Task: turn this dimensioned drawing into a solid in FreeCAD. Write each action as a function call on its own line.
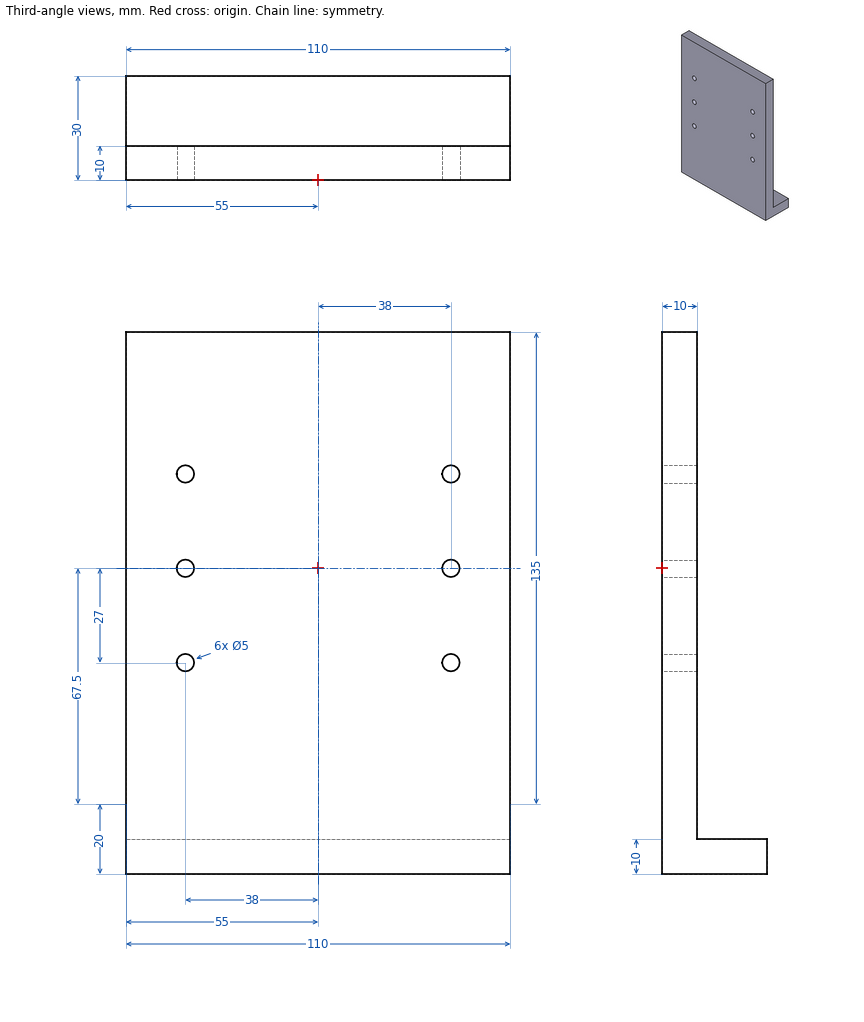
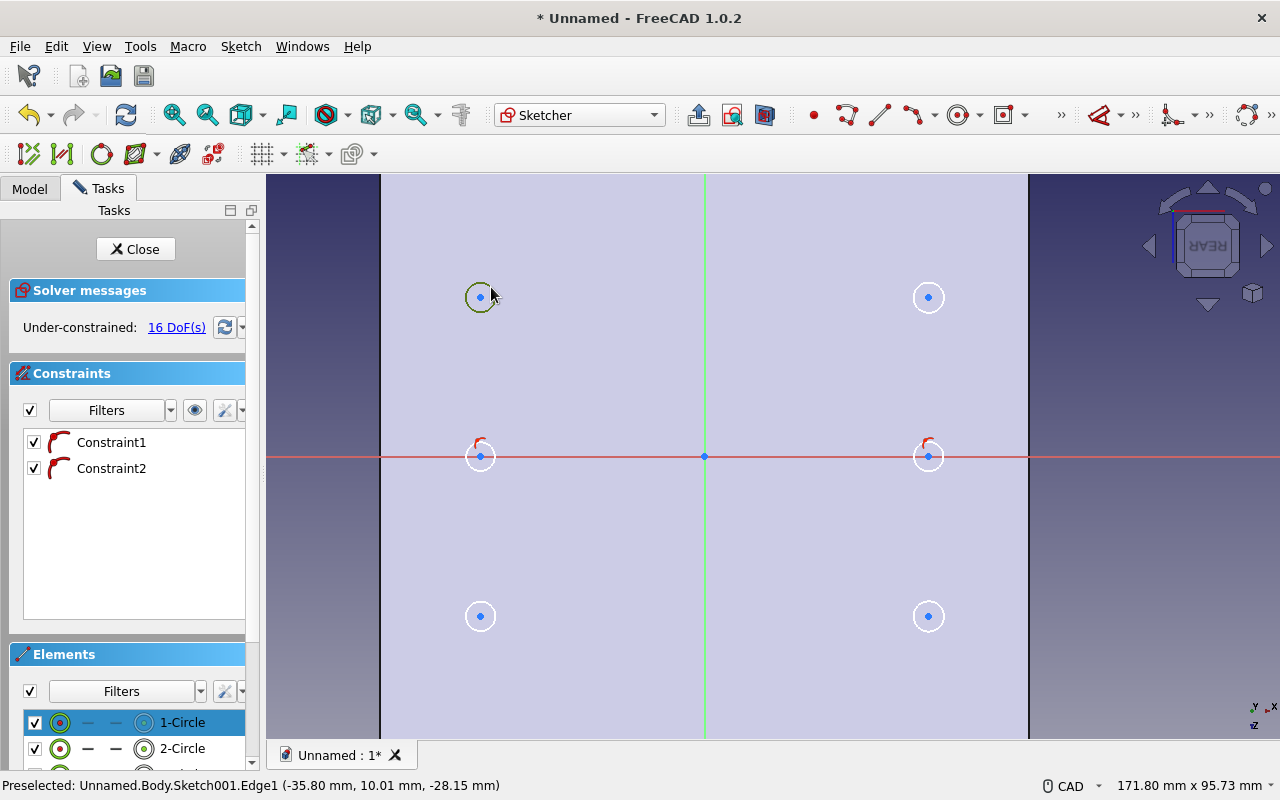
scroll(491, 446, up, 2)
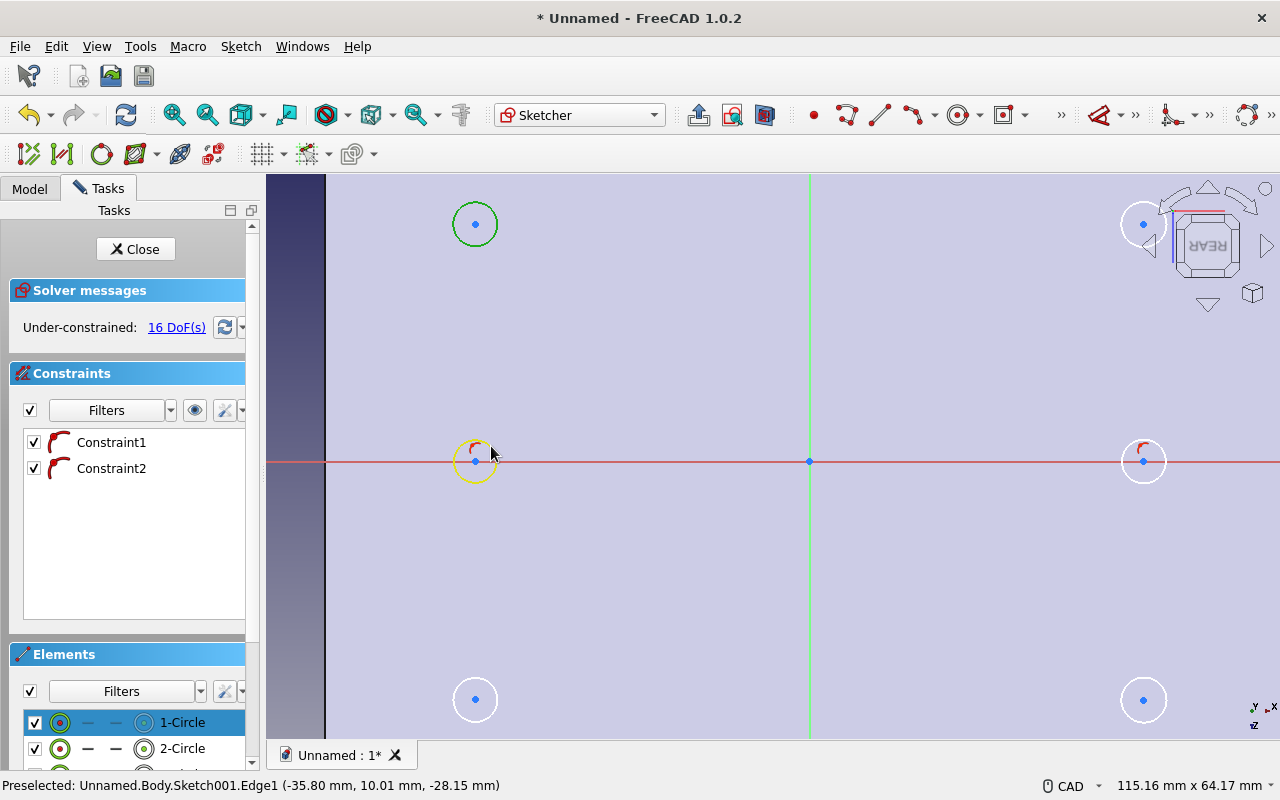
click(490, 446)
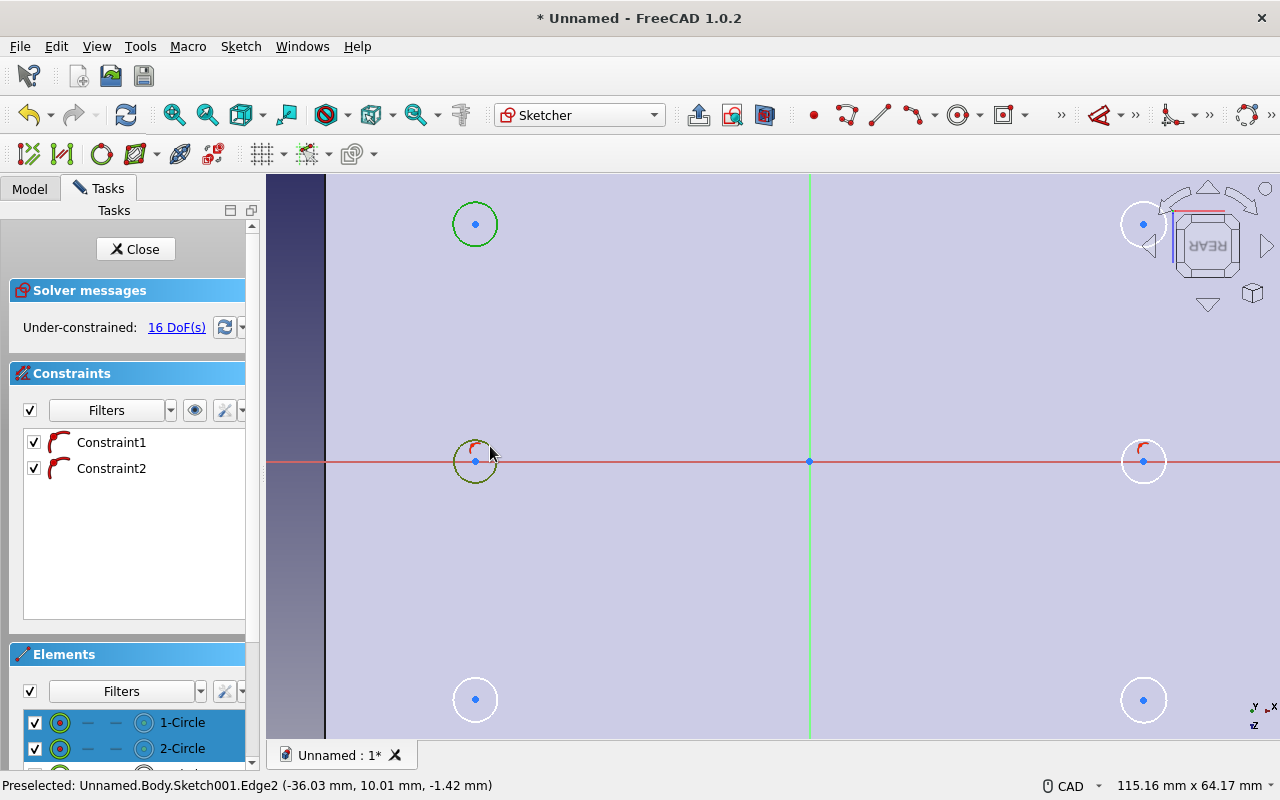
scroll(491, 446, down, 2)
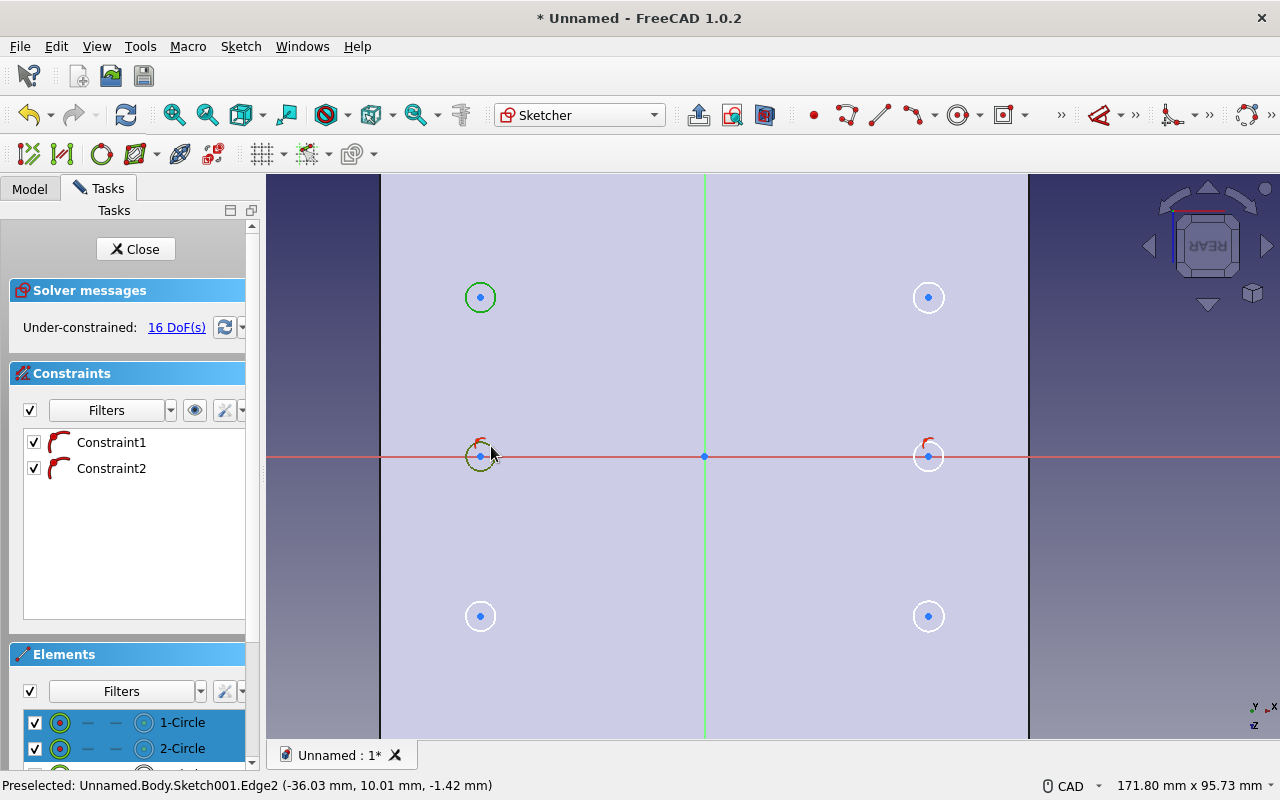
scroll(939, 446, up, 2)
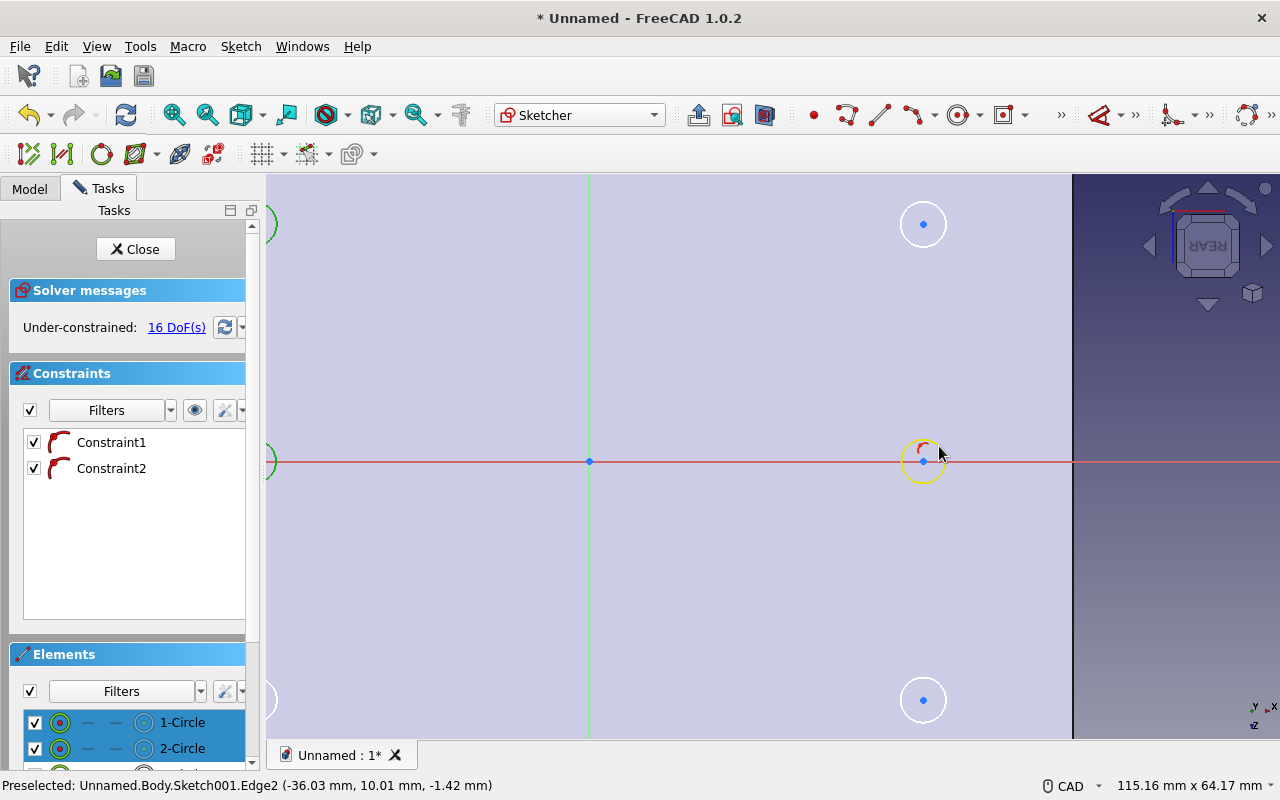
click(939, 446)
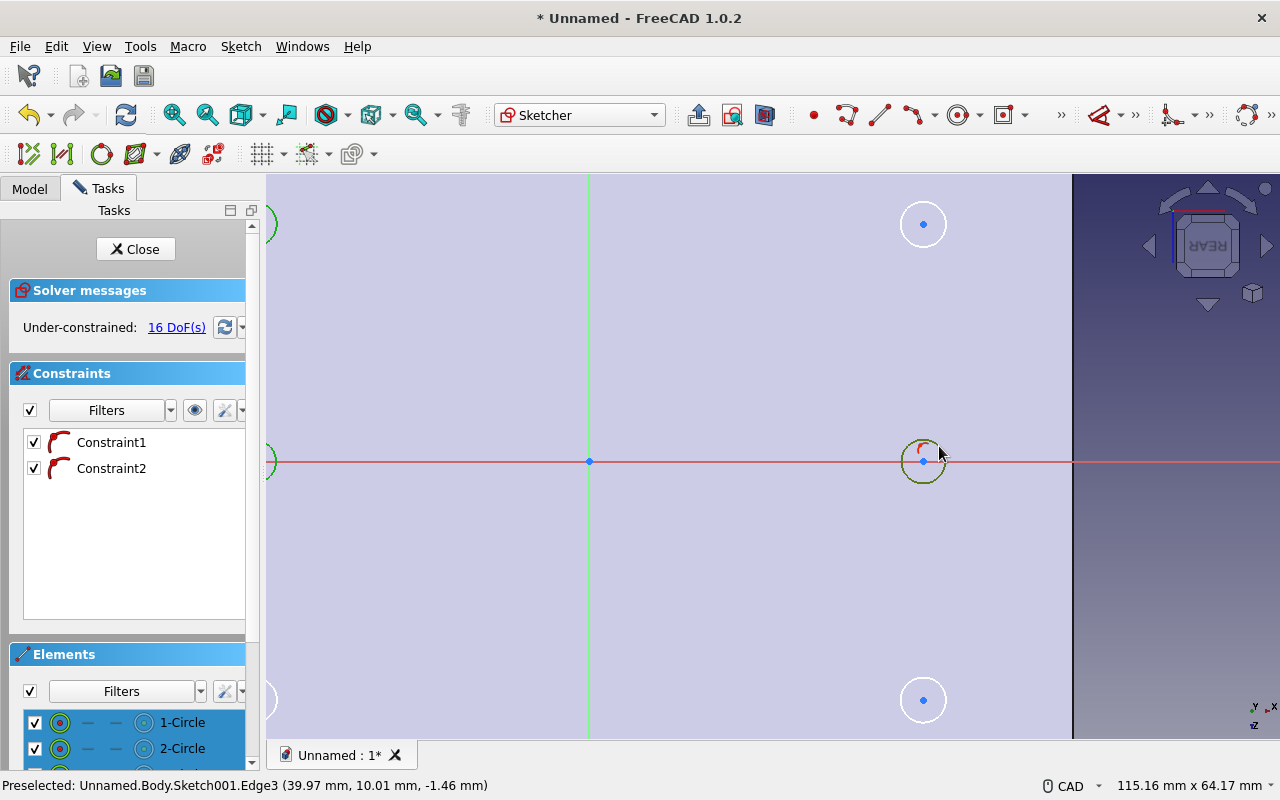
scroll(939, 446, down, 2)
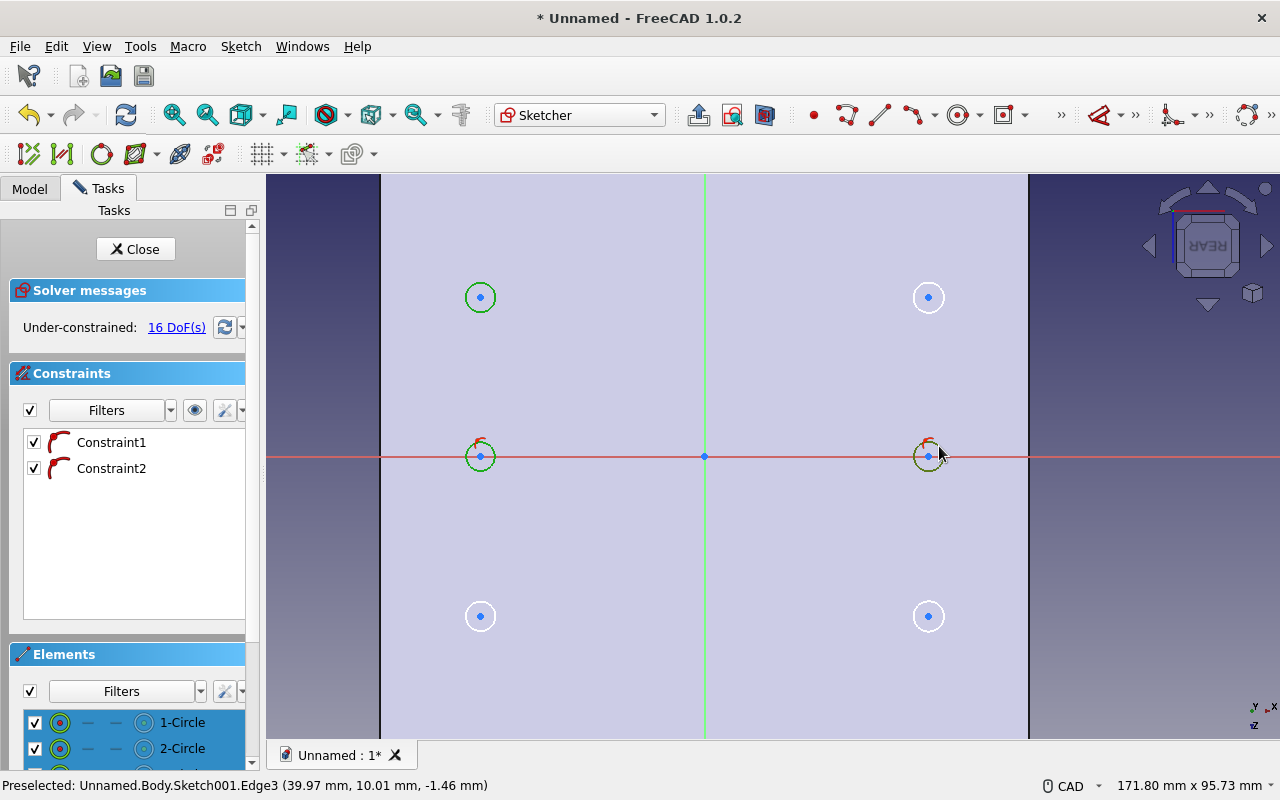
click(491, 606)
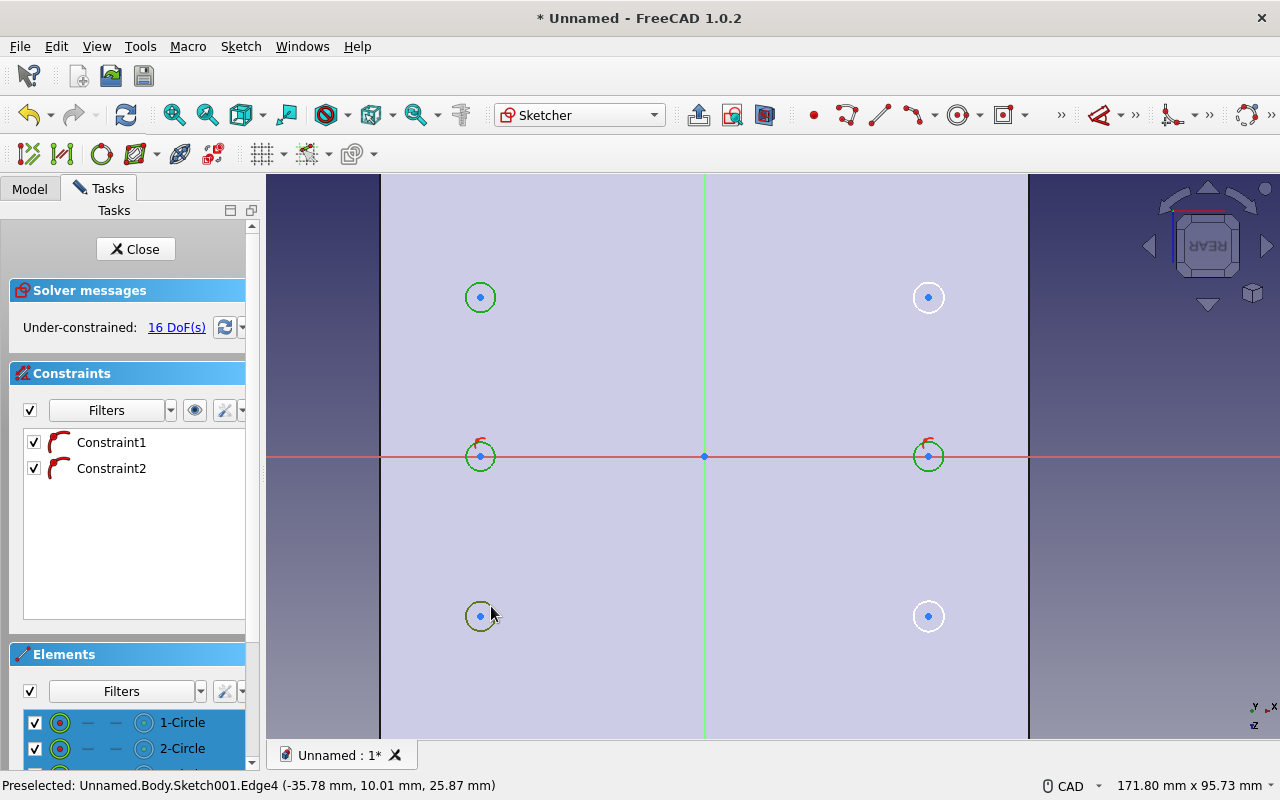
click(939, 606)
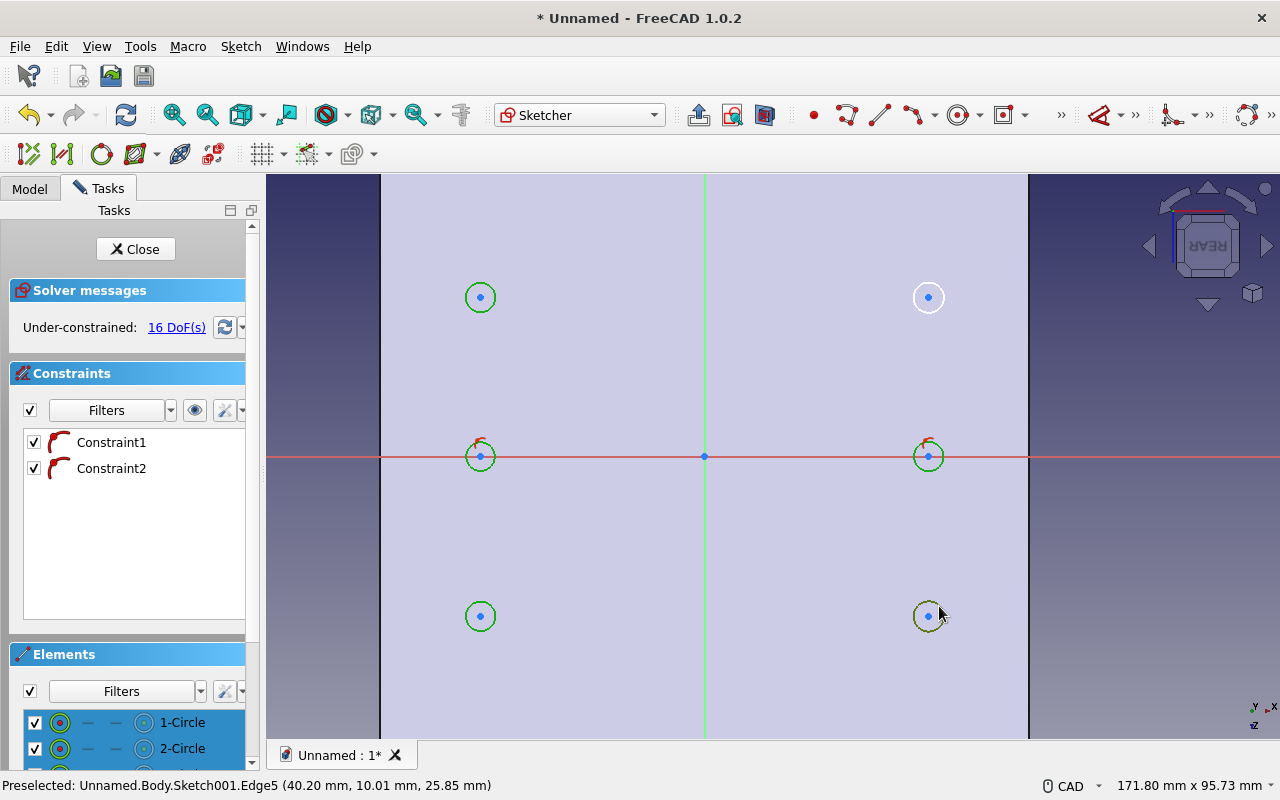
click(939, 287)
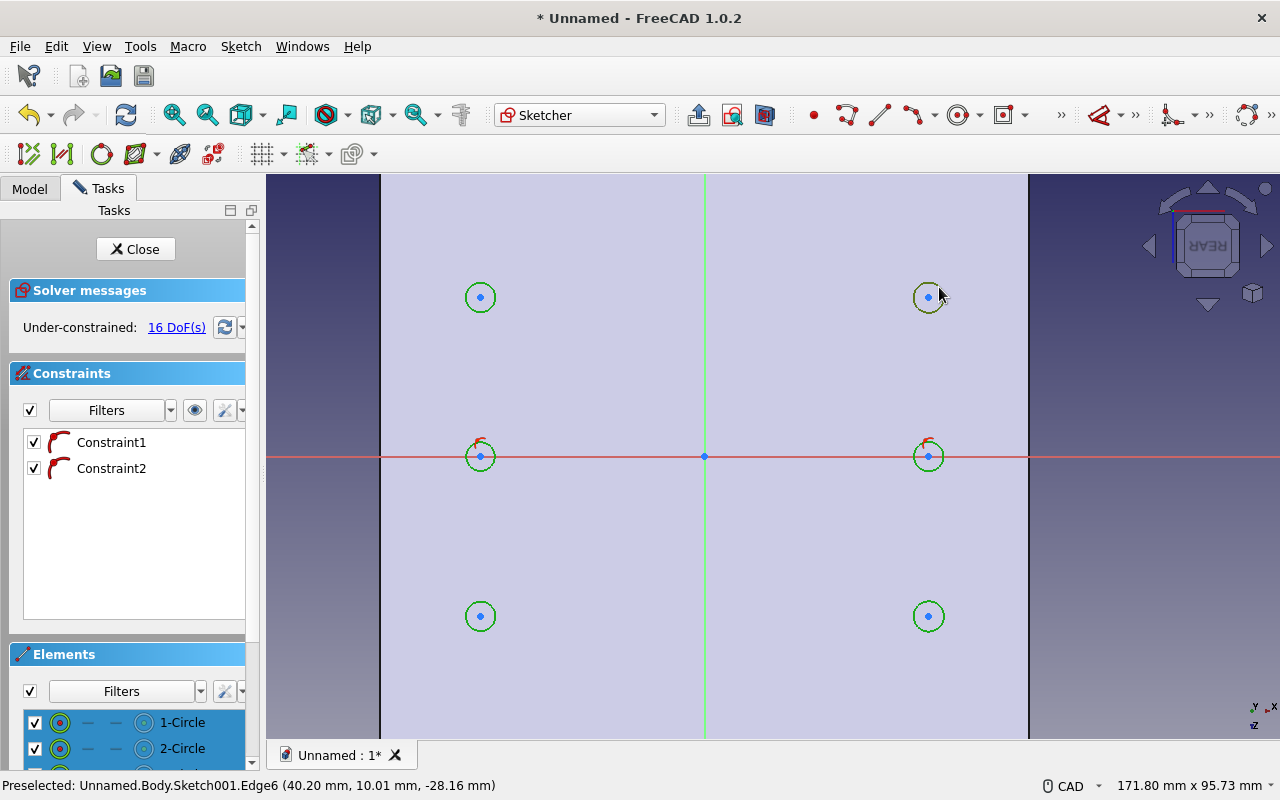
key(e)